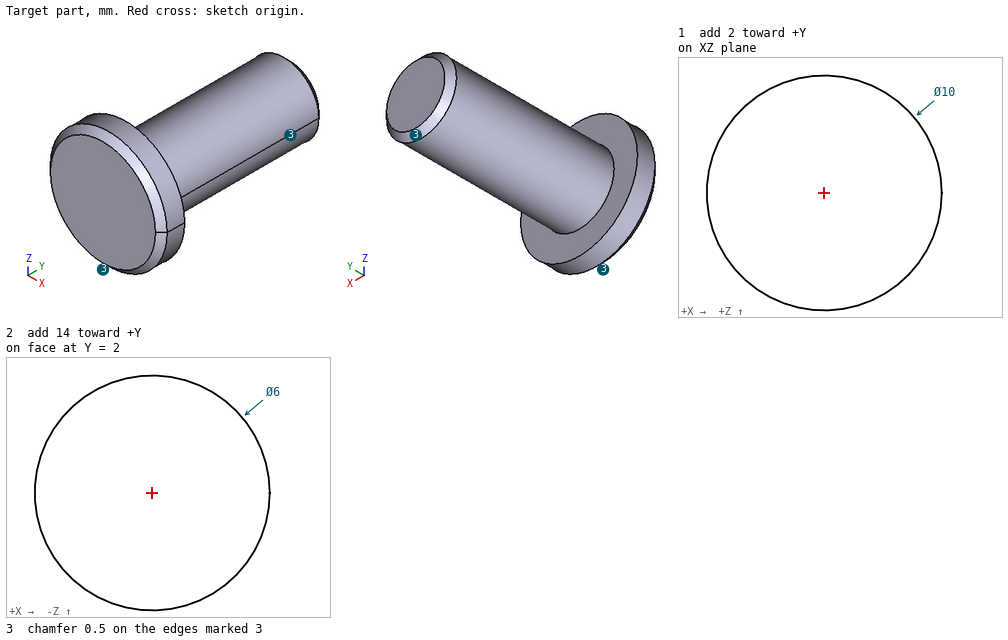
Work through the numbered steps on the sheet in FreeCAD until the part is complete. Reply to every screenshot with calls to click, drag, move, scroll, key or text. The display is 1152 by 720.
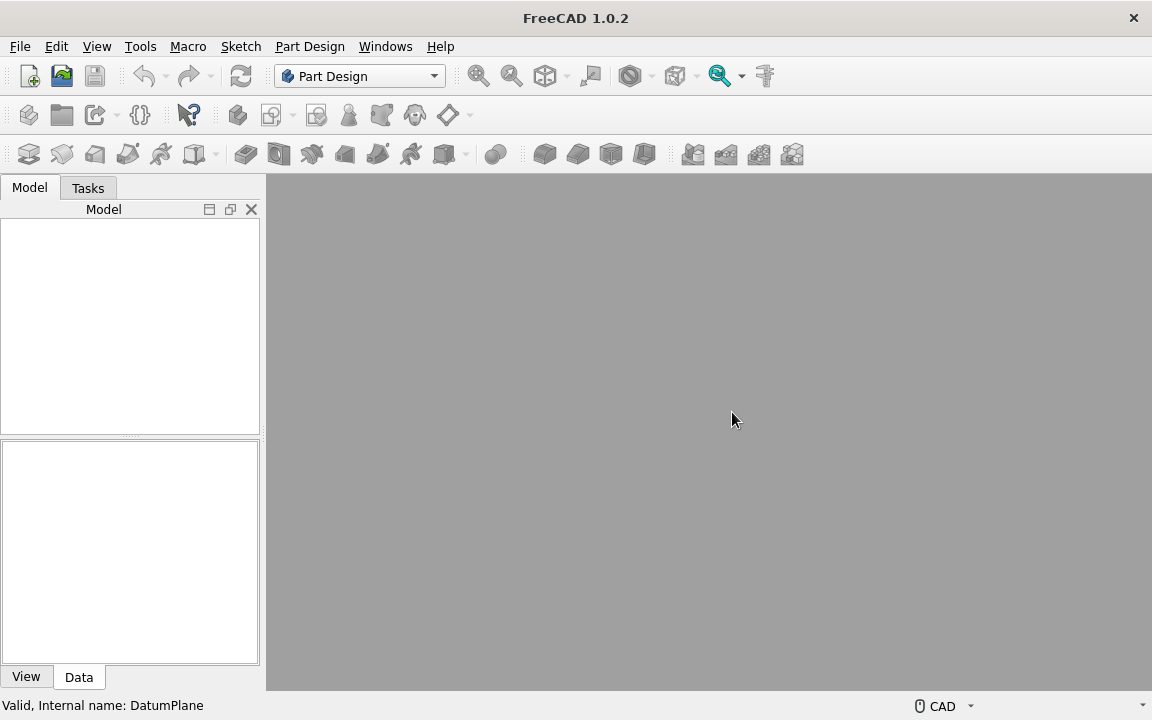
click(29, 76)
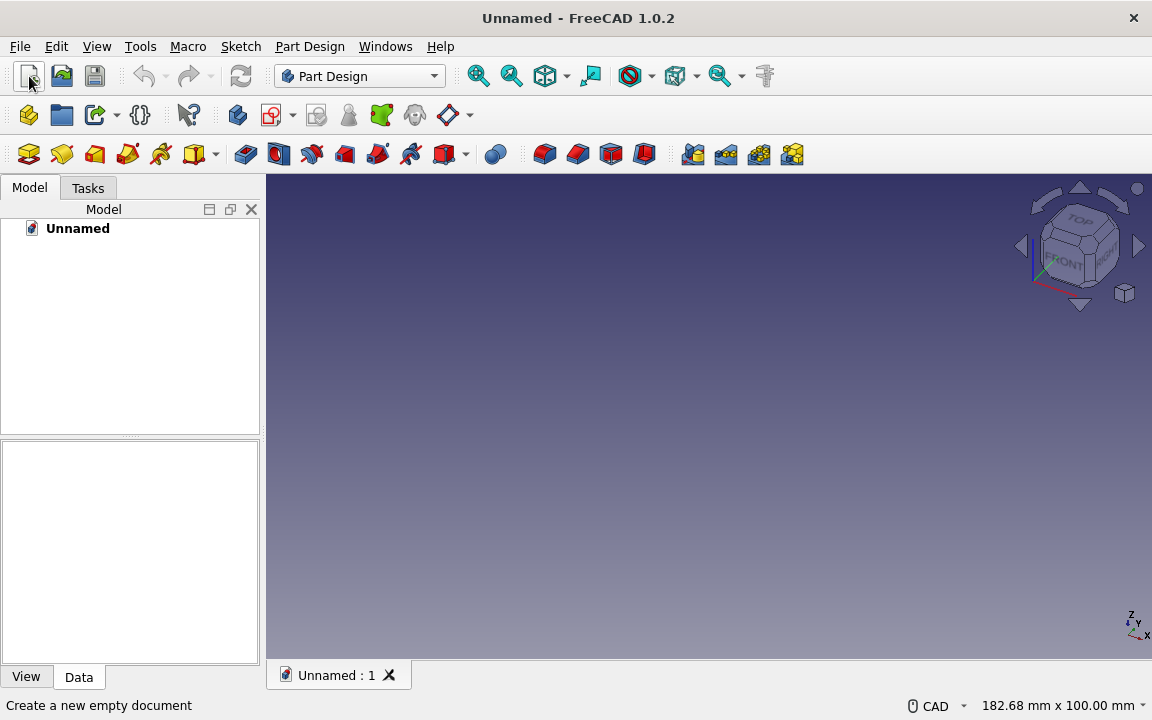
click(270, 116)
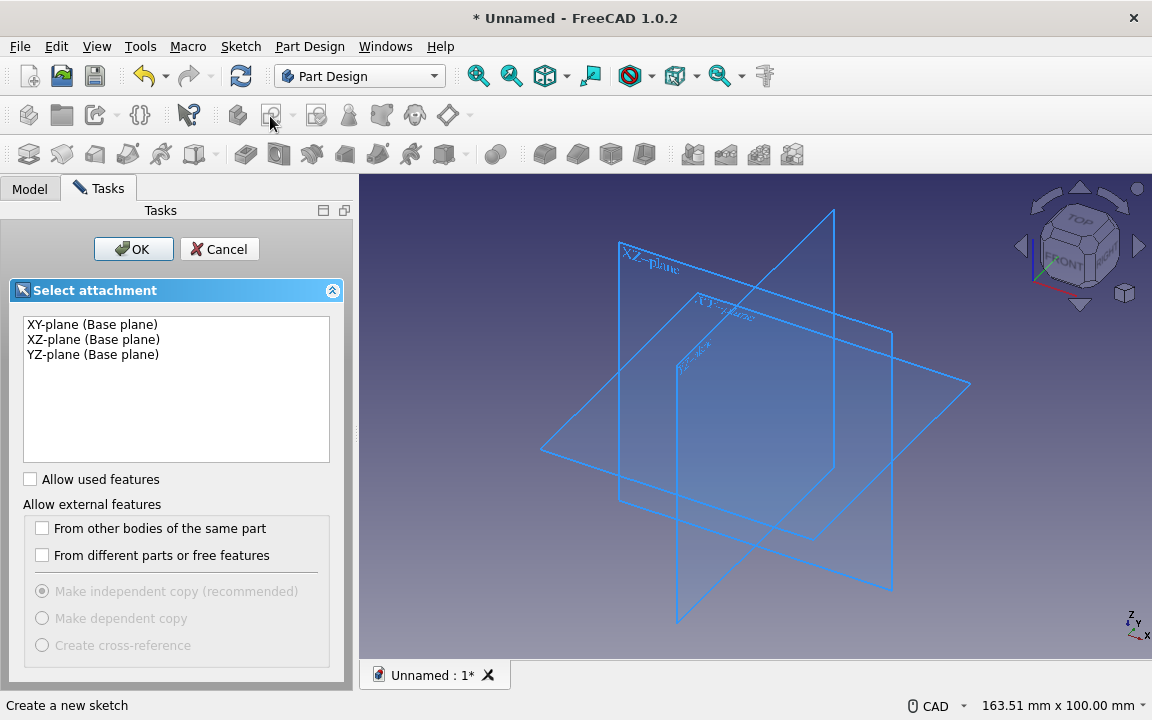
click(84, 340)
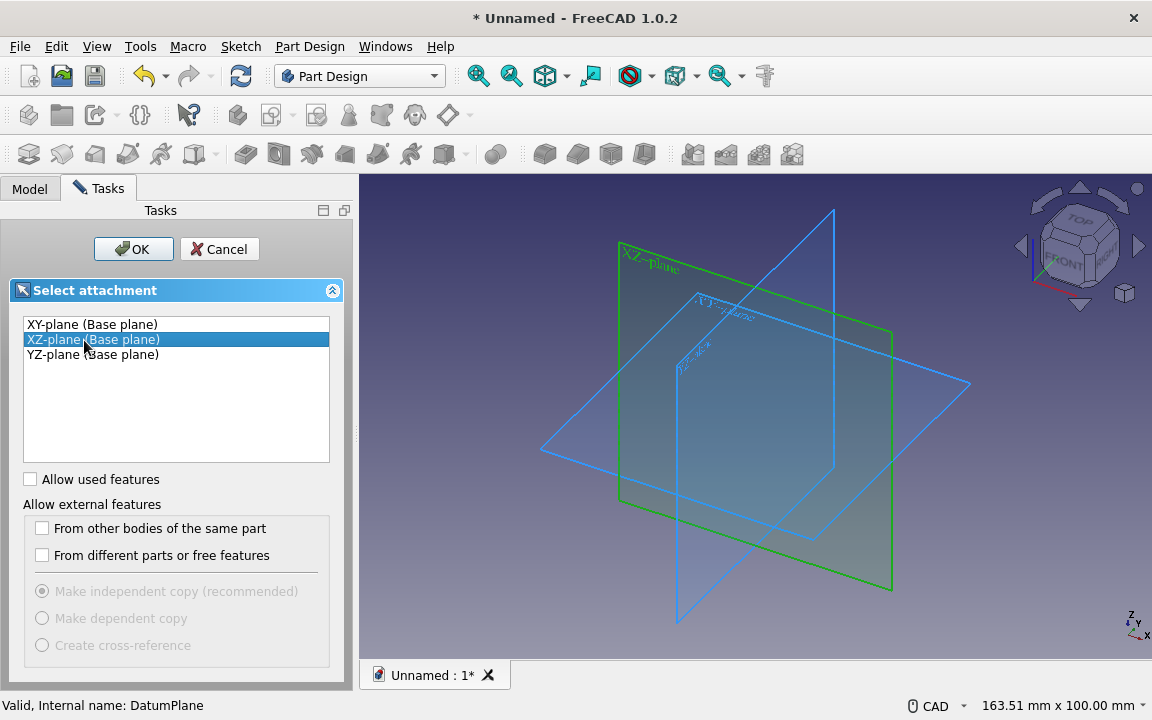
click(134, 249)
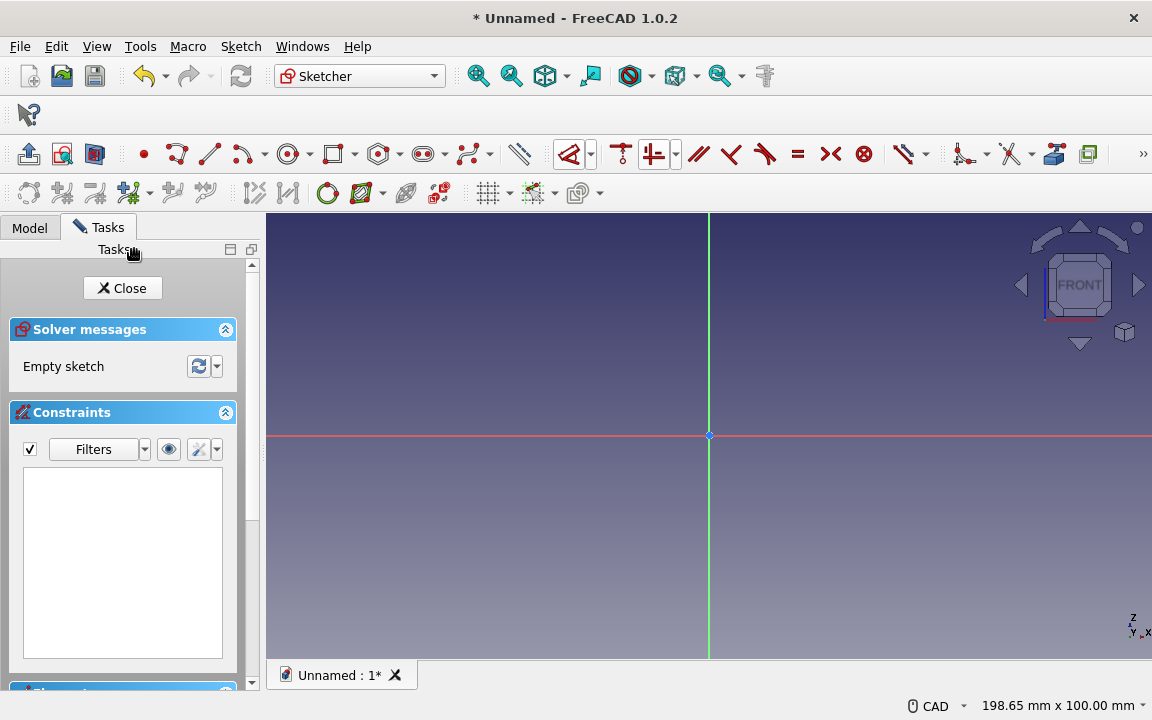
scroll(723, 436, up, 9)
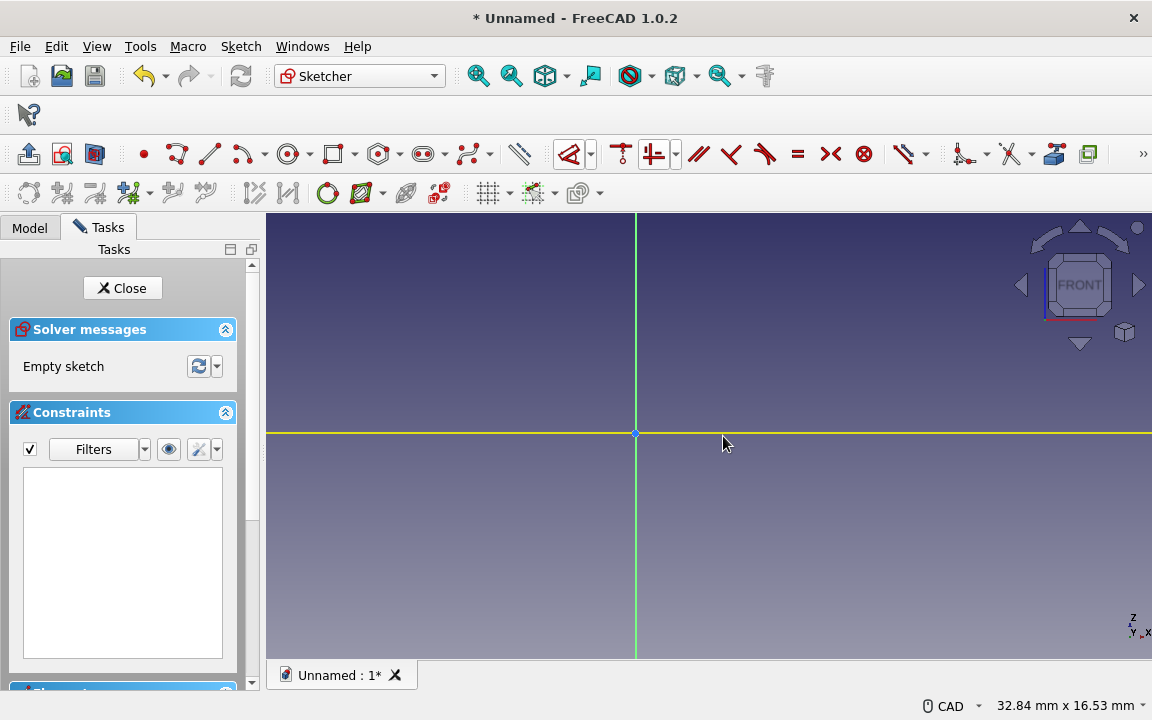
click(288, 154)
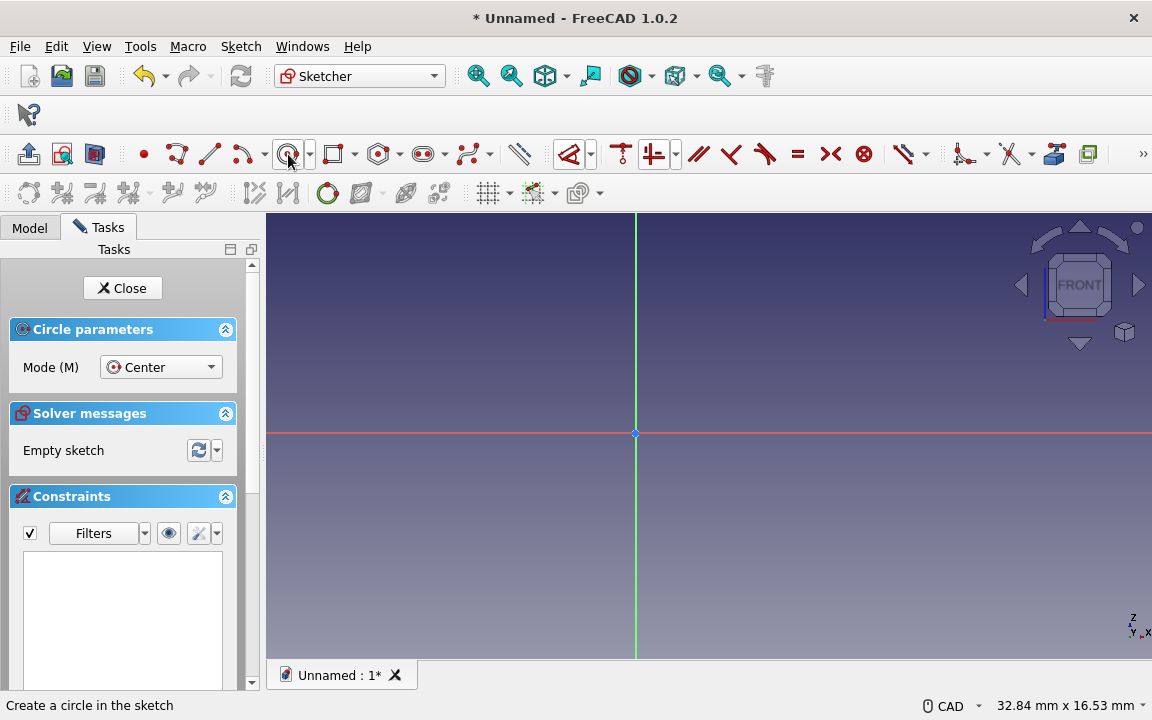
click(636, 433)
click(731, 338)
key(Escape)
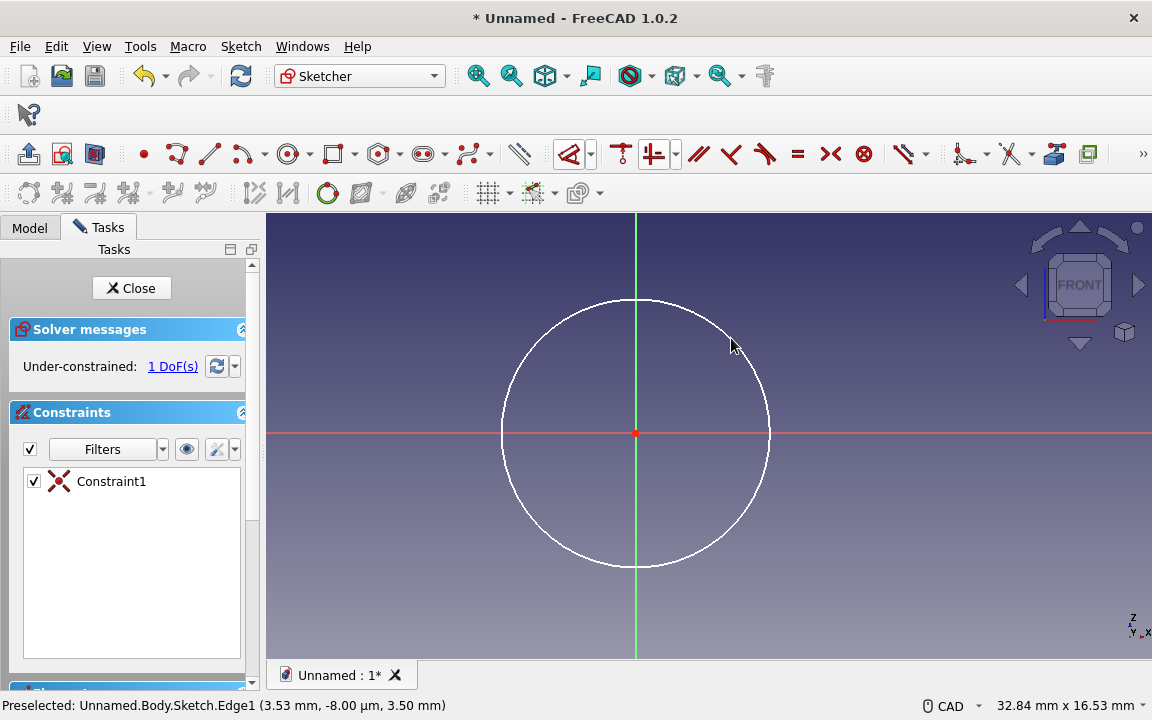
key(d)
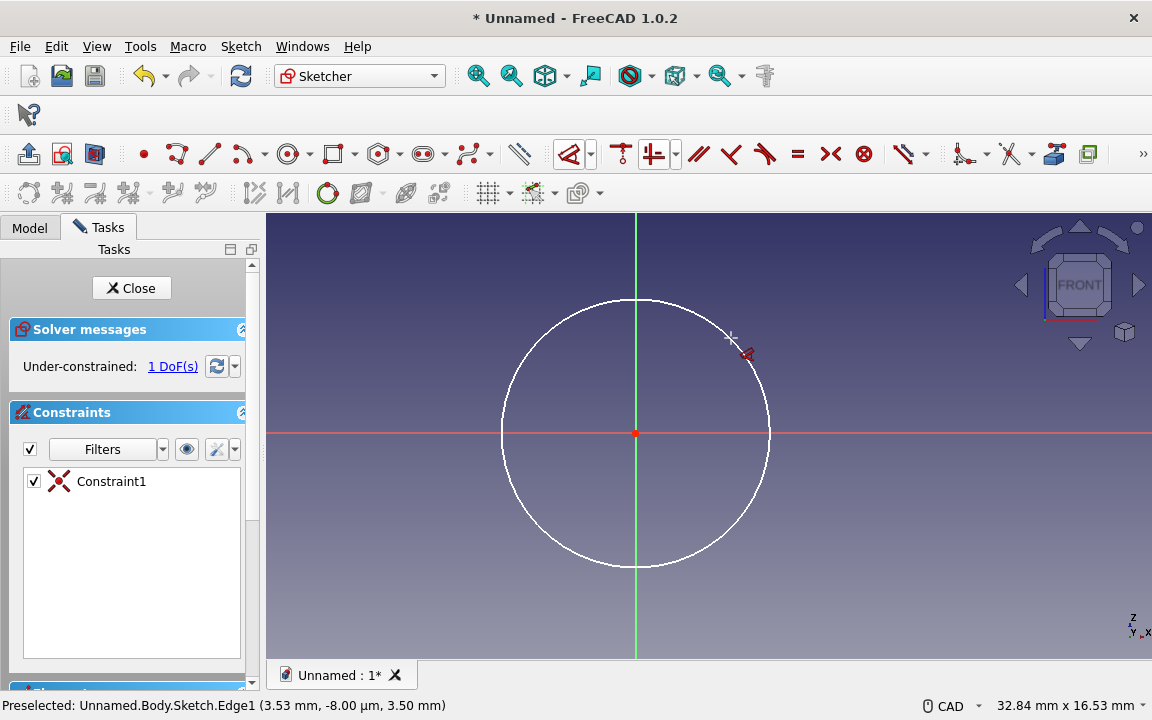
click(730, 338)
click(752, 315)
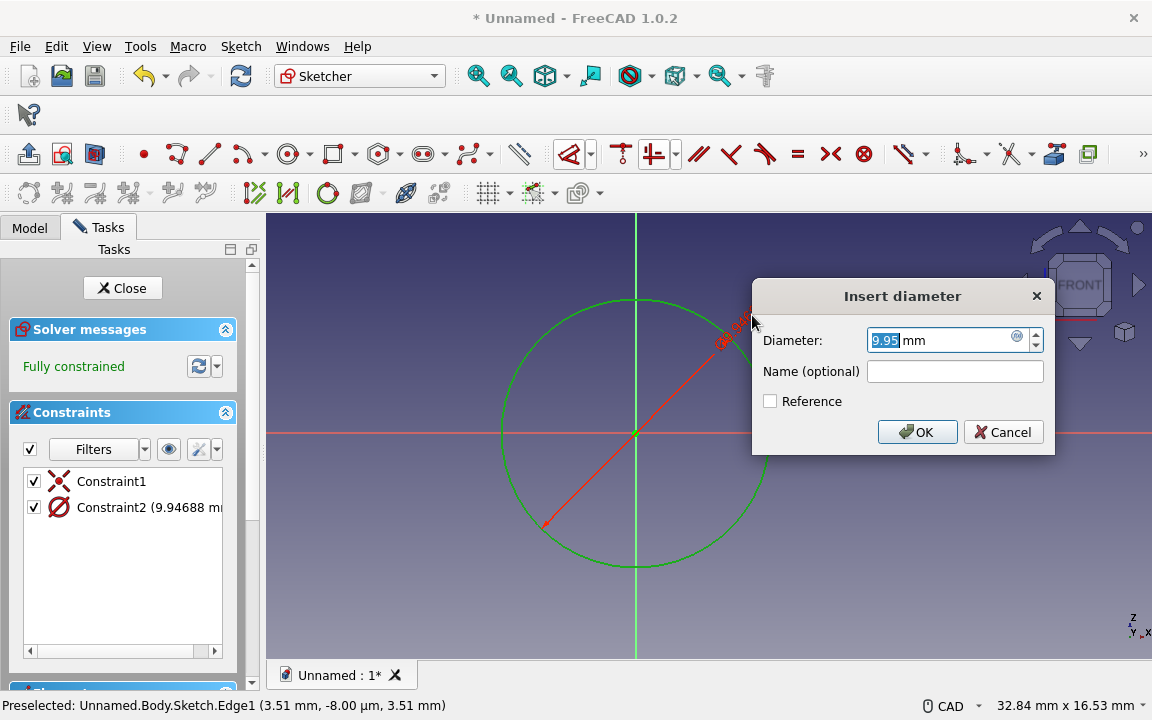
text(10)
key(Return)
key(Escape)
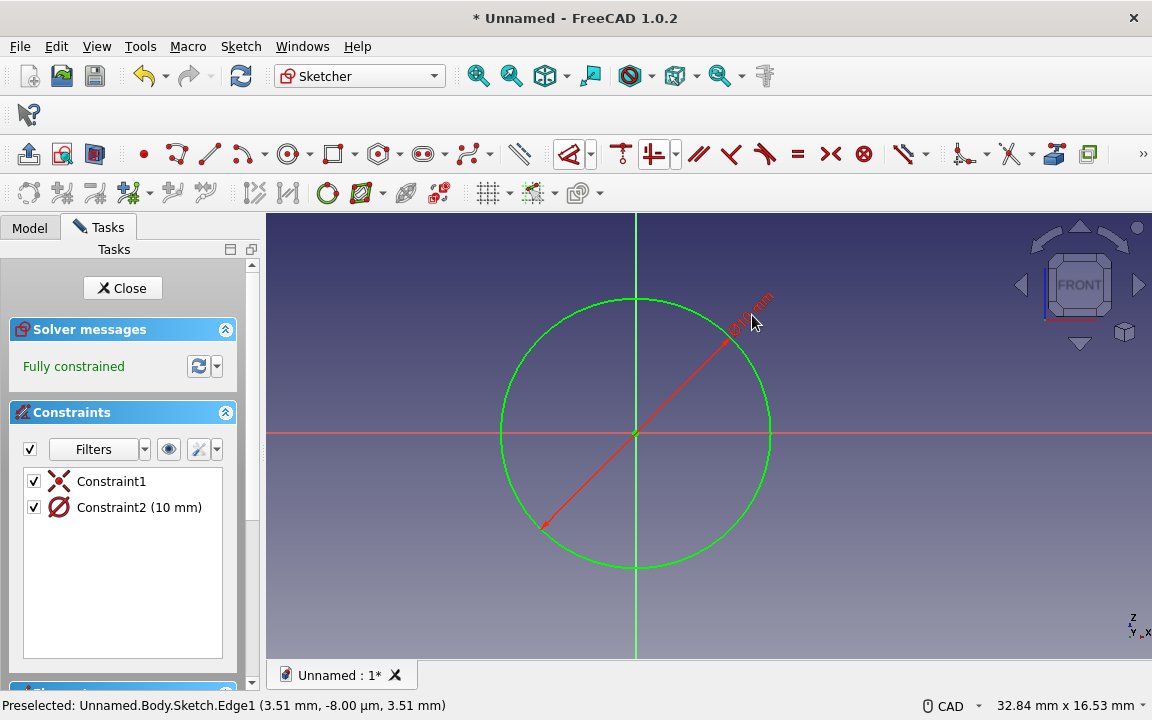
click(123, 288)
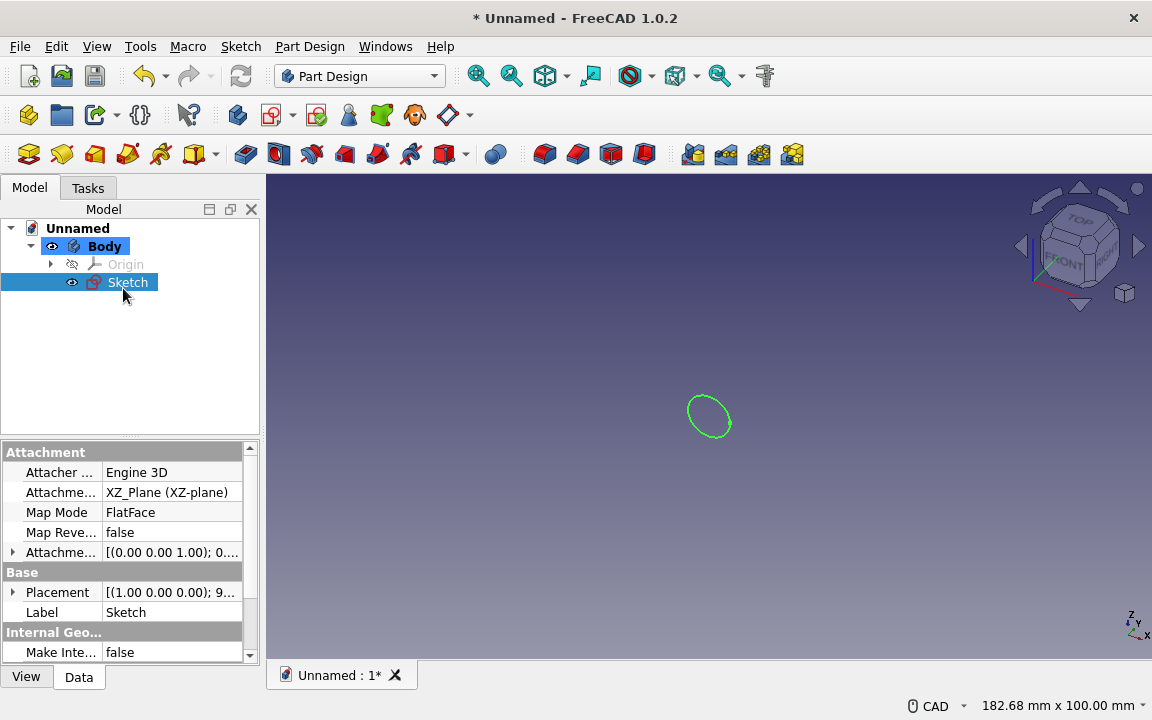
click(29, 154)